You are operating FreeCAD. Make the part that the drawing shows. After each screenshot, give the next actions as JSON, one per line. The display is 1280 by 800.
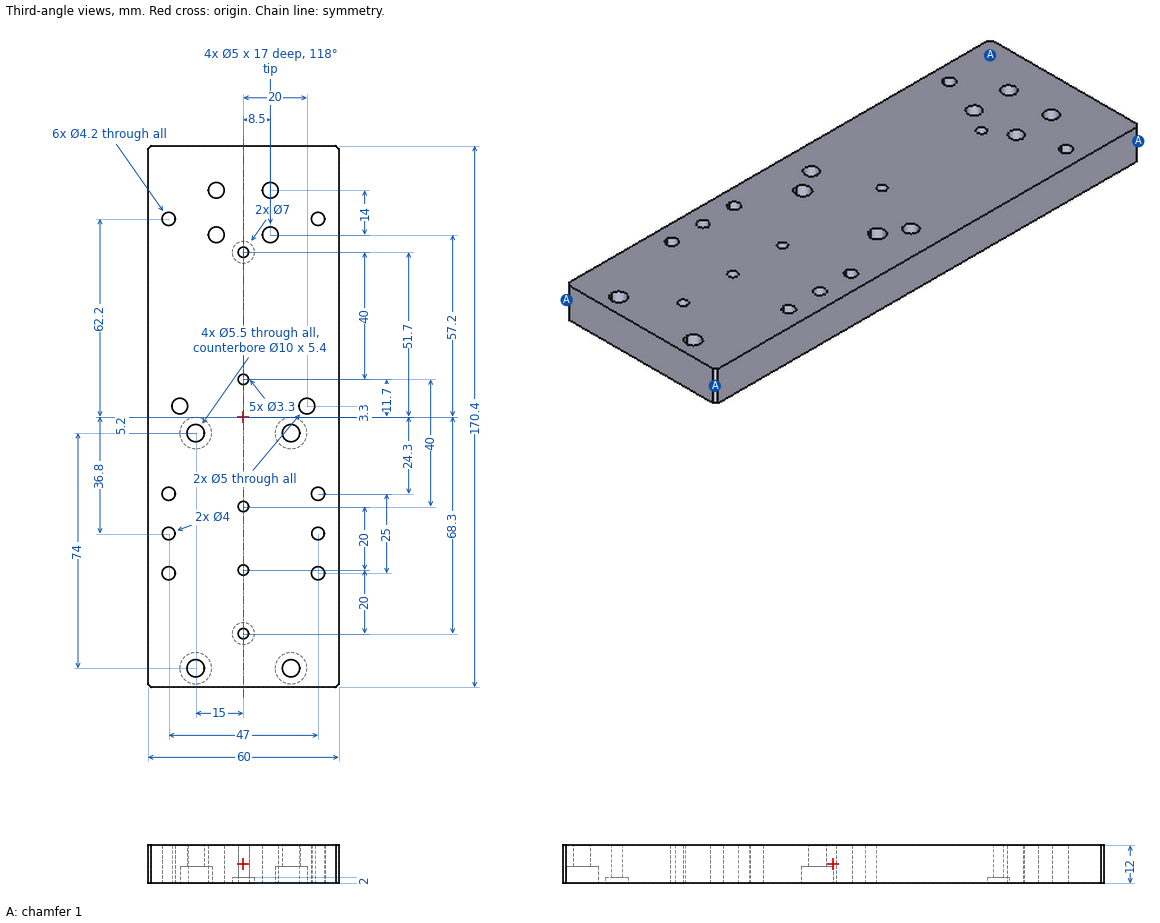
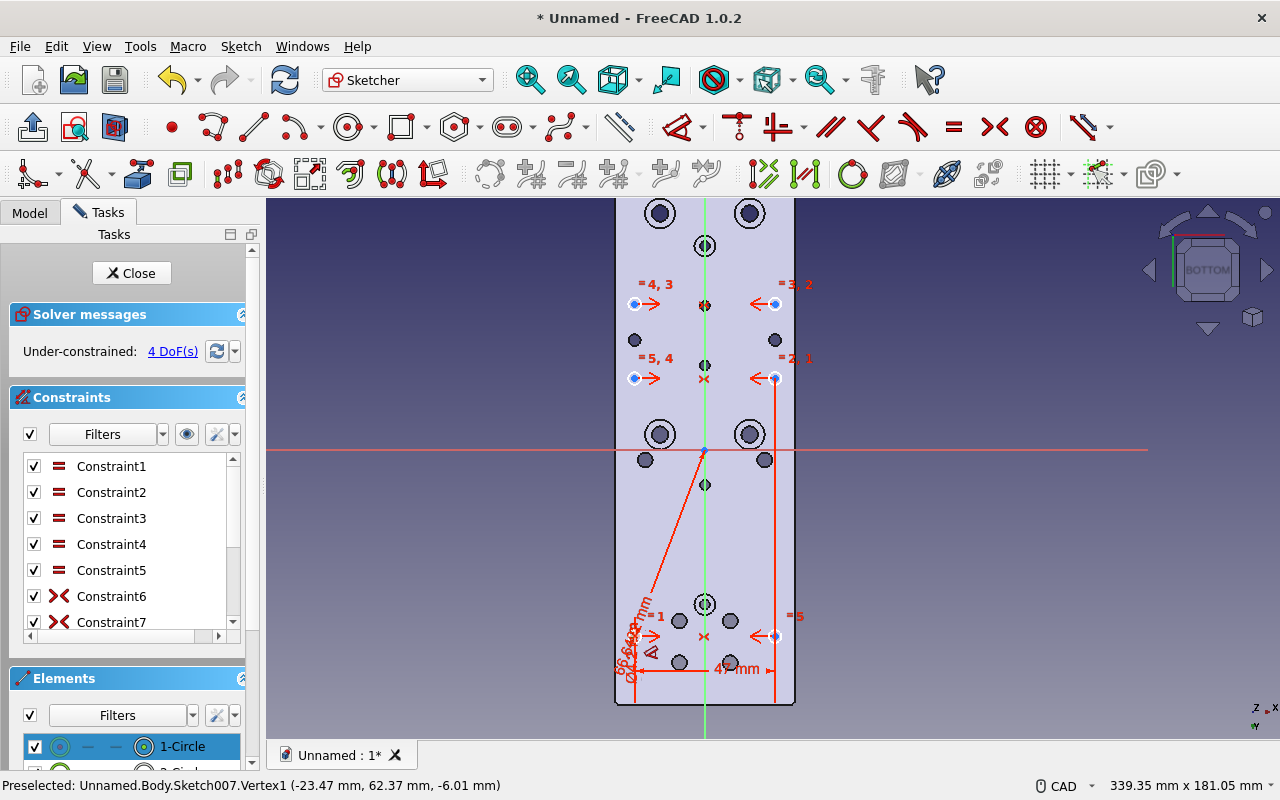
{"action": "left_click", "coordinate": [775, 304]}
{"action": "left_click", "coordinate": [673, 270]}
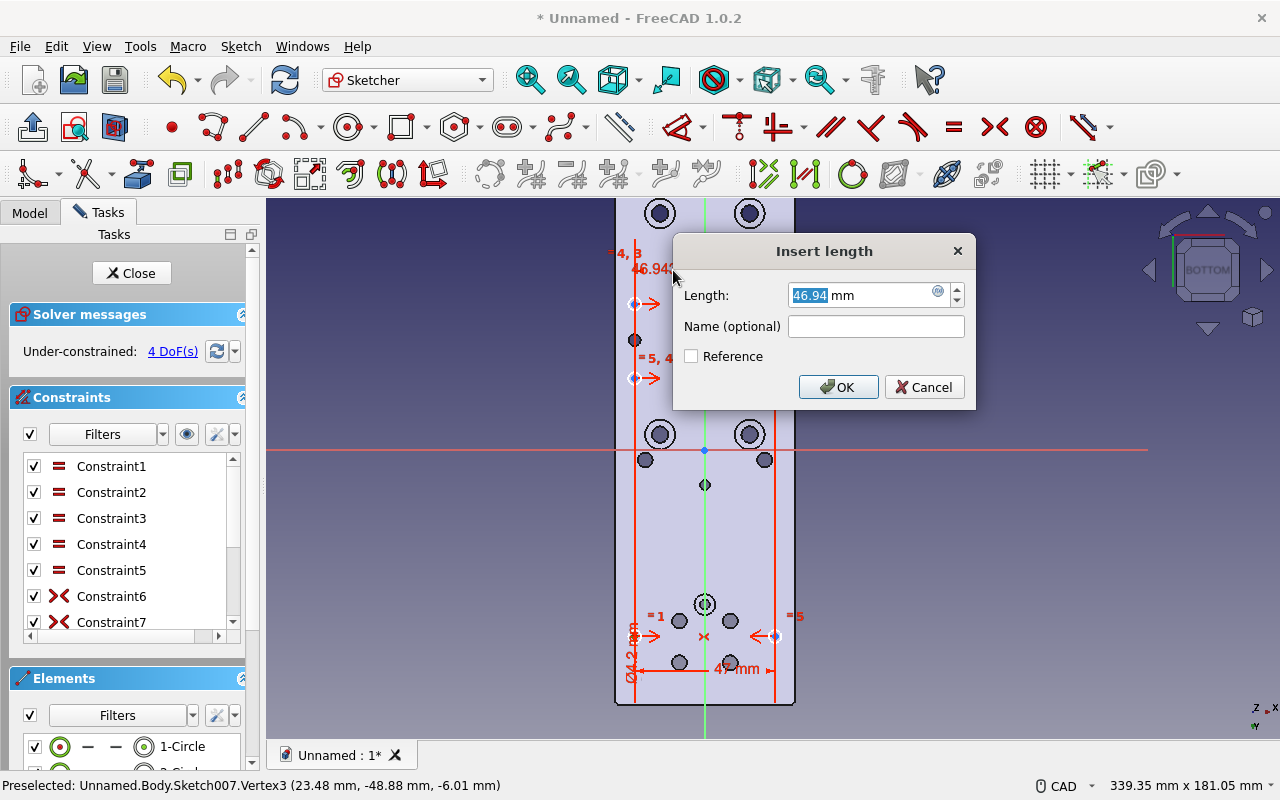
{"action": "type", "text": "47"}
{"action": "key", "text": "Return"}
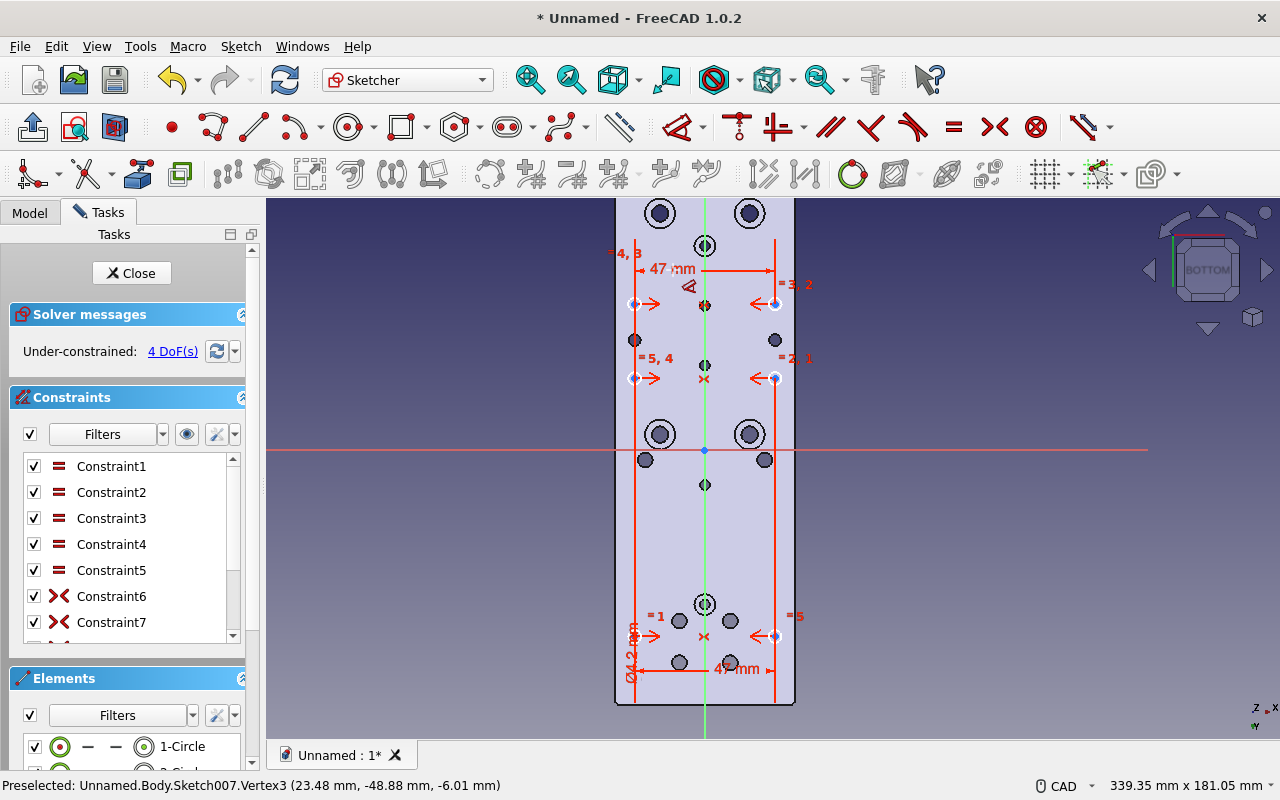
{"action": "left_click", "coordinate": [775, 378]}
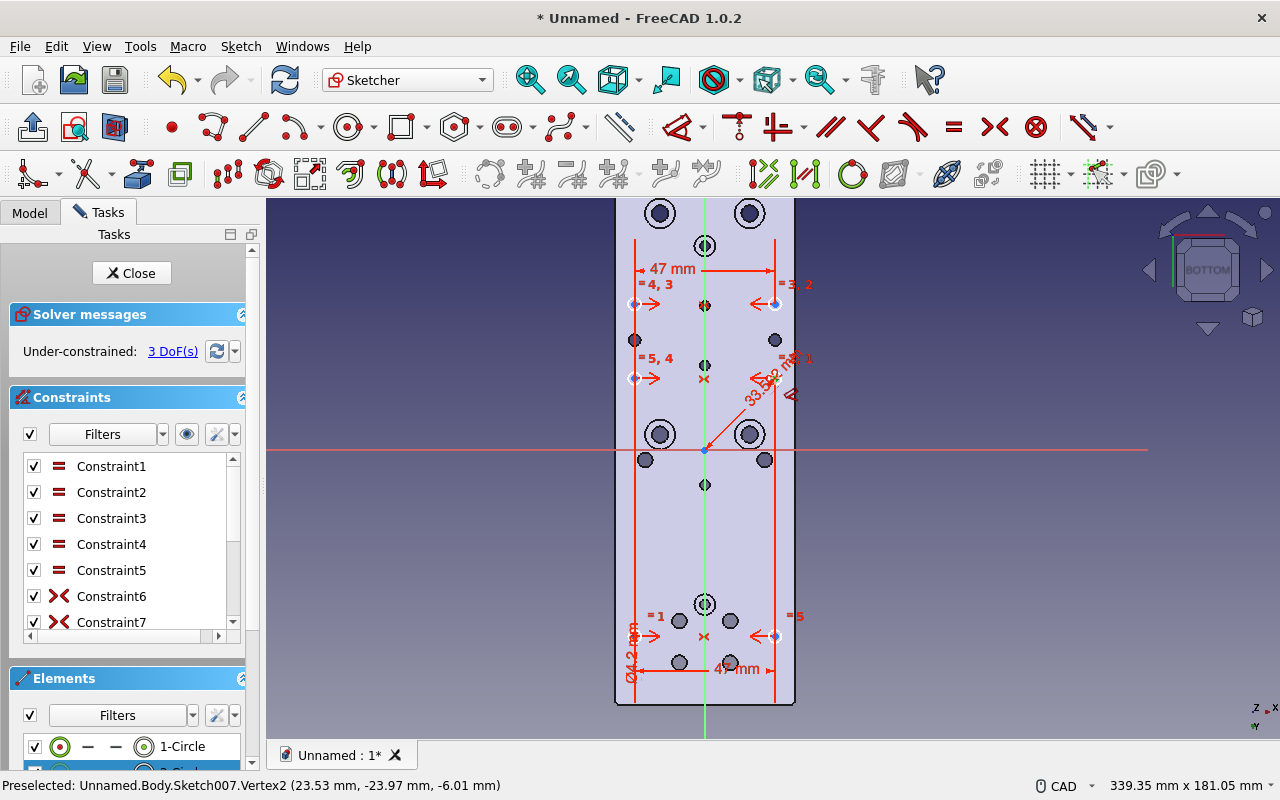
{"action": "left_click", "coordinate": [775, 304]}
{"action": "left_click", "coordinate": [809, 341]}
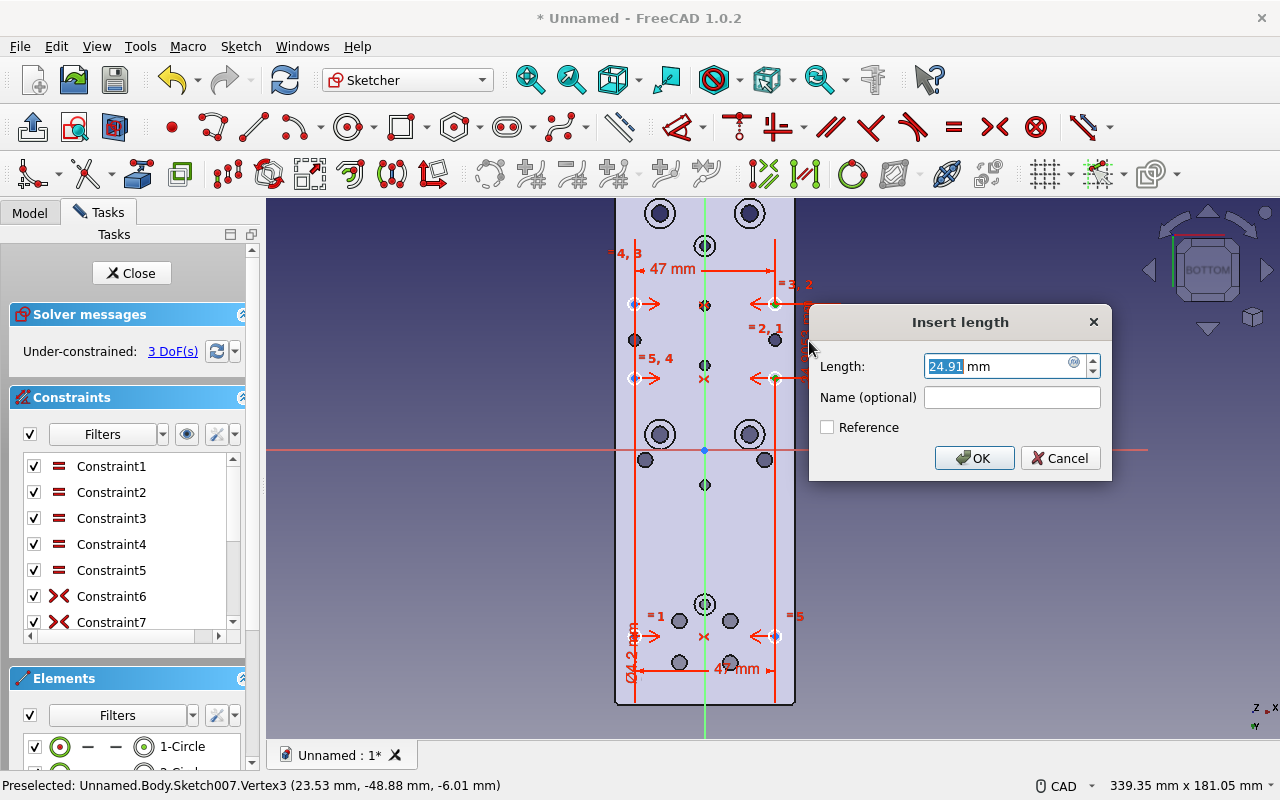
{"action": "type", "text": "25"}
{"action": "key", "text": "Return"}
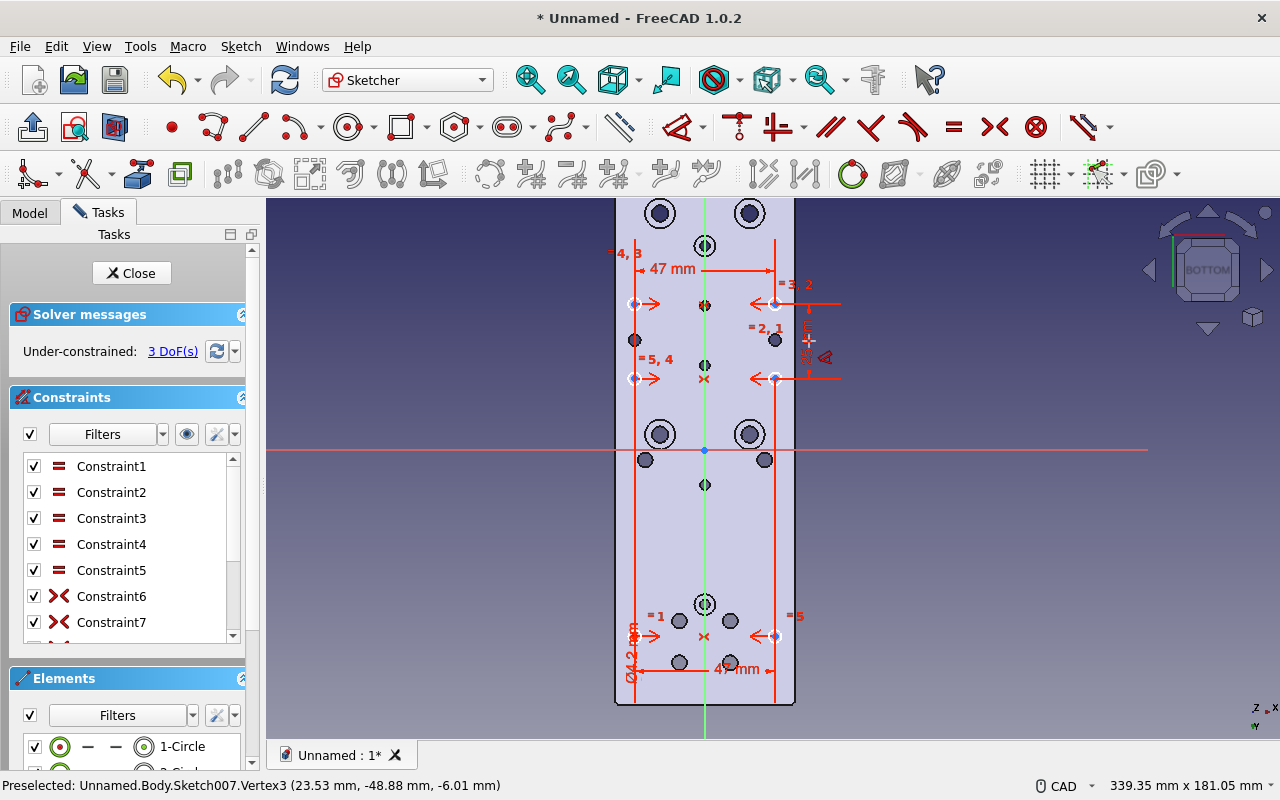
{"action": "left_click", "coordinate": [775, 304]}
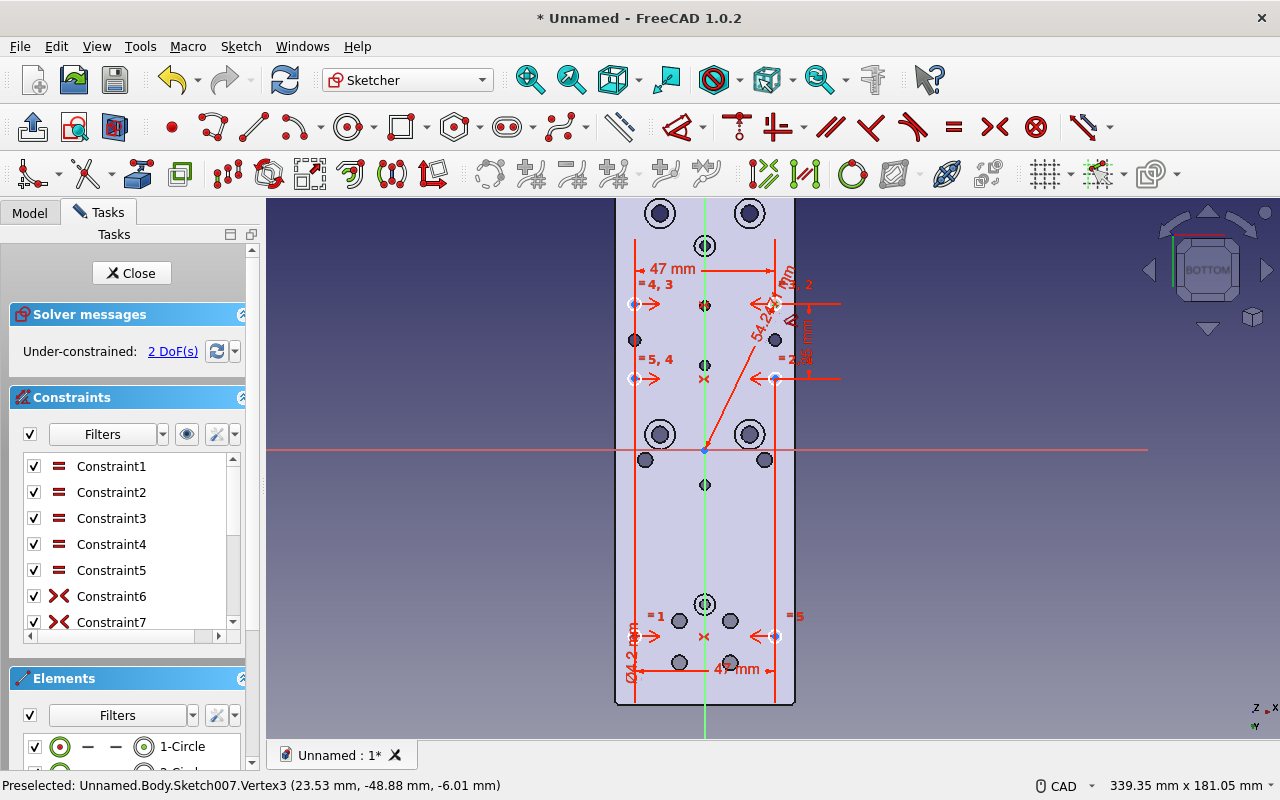
{"action": "left_click", "coordinate": [635, 304]}
{"action": "left_click", "coordinate": [754, 270]}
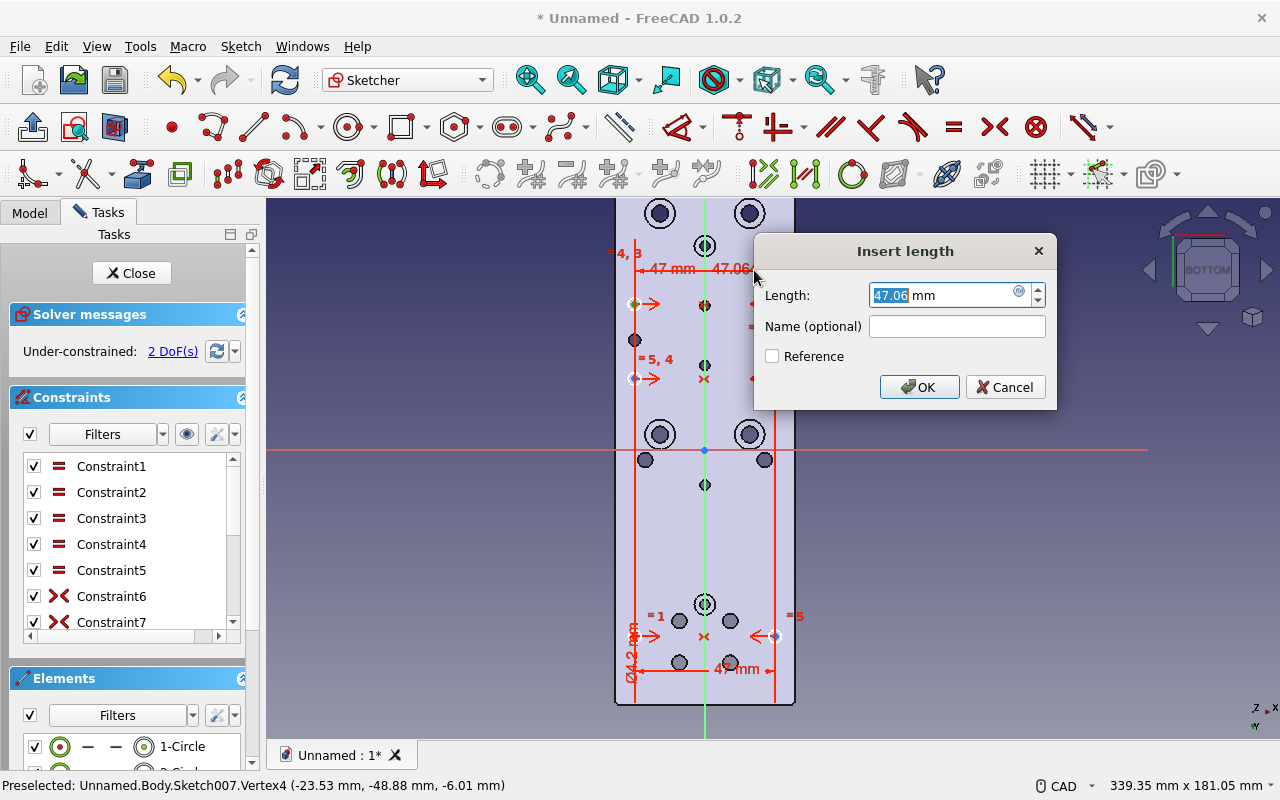
{"action": "type", "text": "47"}
{"action": "key", "text": "Return"}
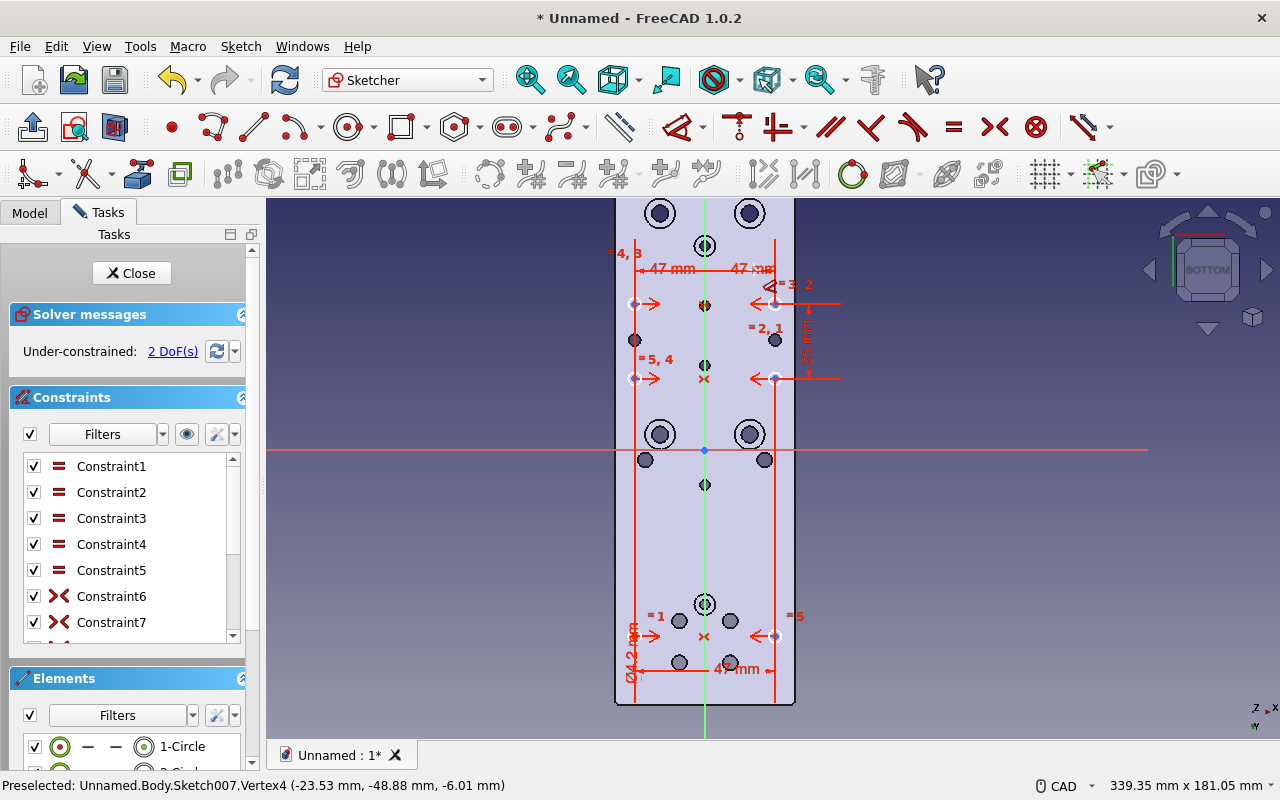
{"action": "left_click", "coordinate": [635, 636]}
{"action": "left_click", "coordinate": [601, 543]}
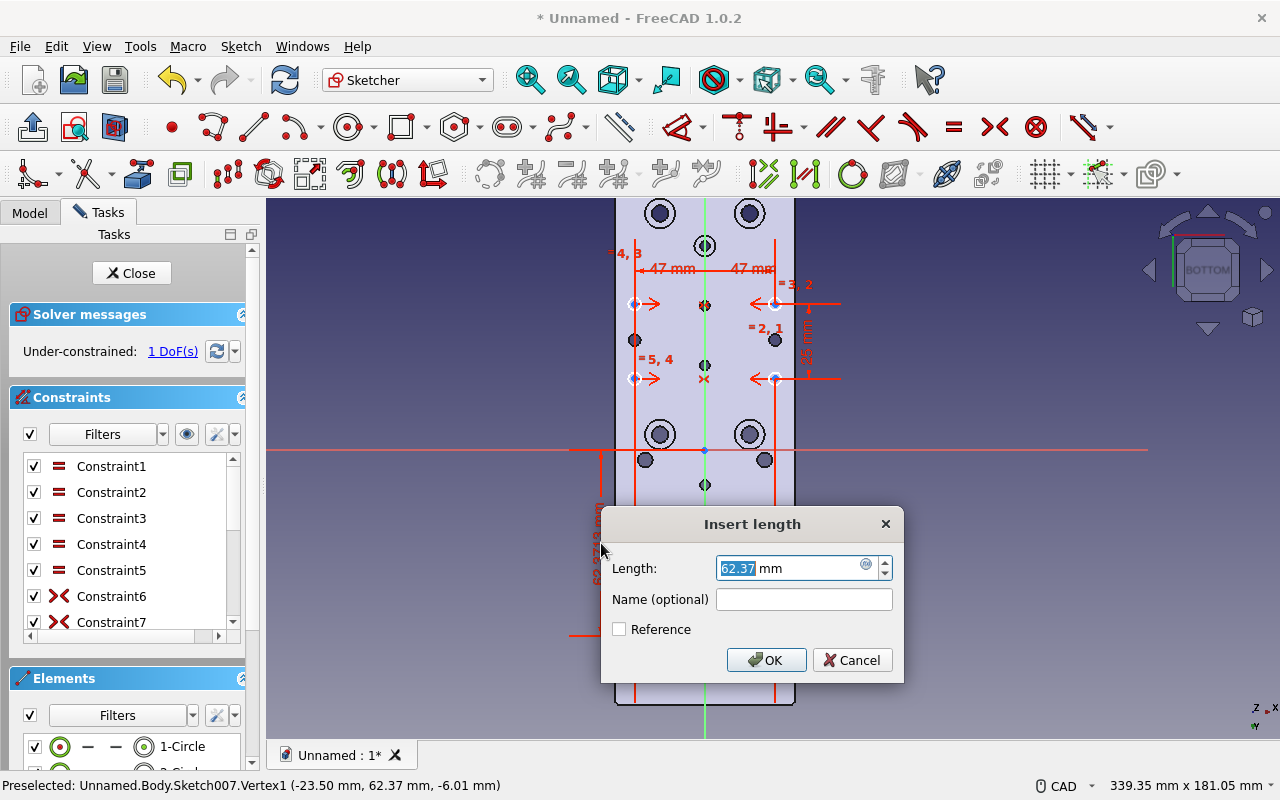
{"action": "type", "text": "62.2"}
{"action": "key", "text": "Return"}